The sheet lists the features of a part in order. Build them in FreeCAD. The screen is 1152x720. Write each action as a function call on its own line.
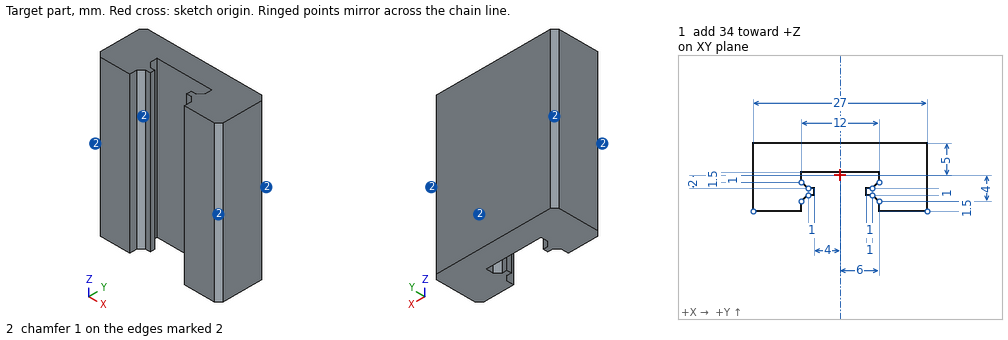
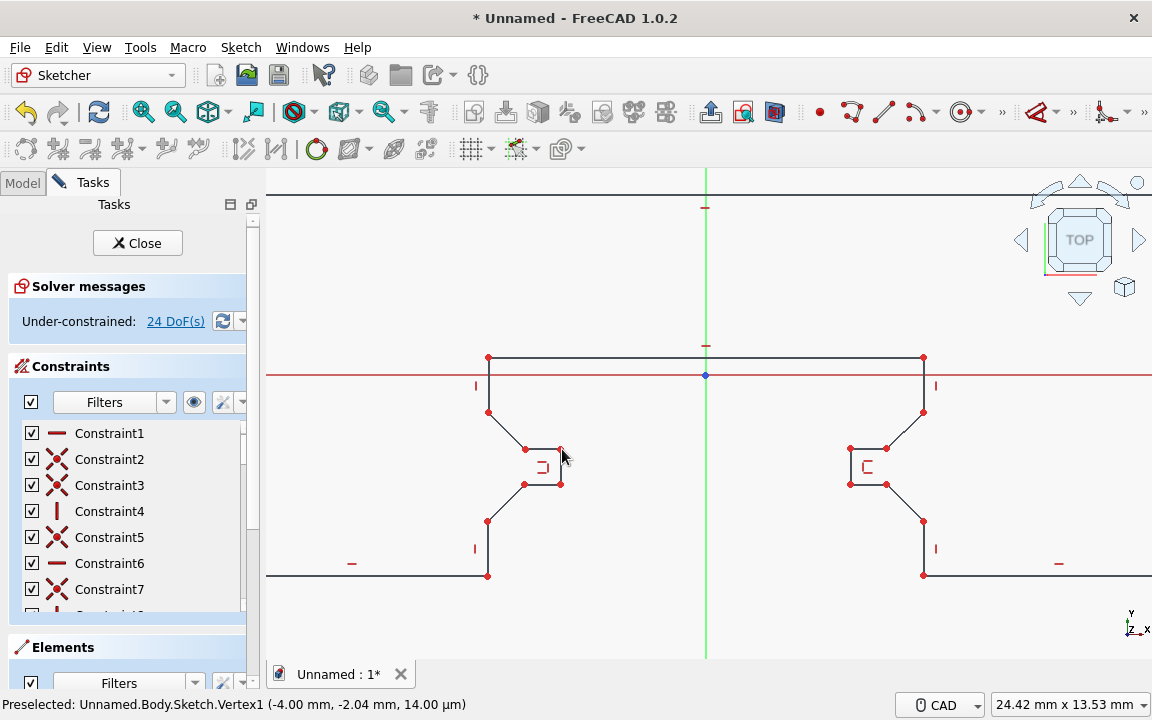
click(489, 413)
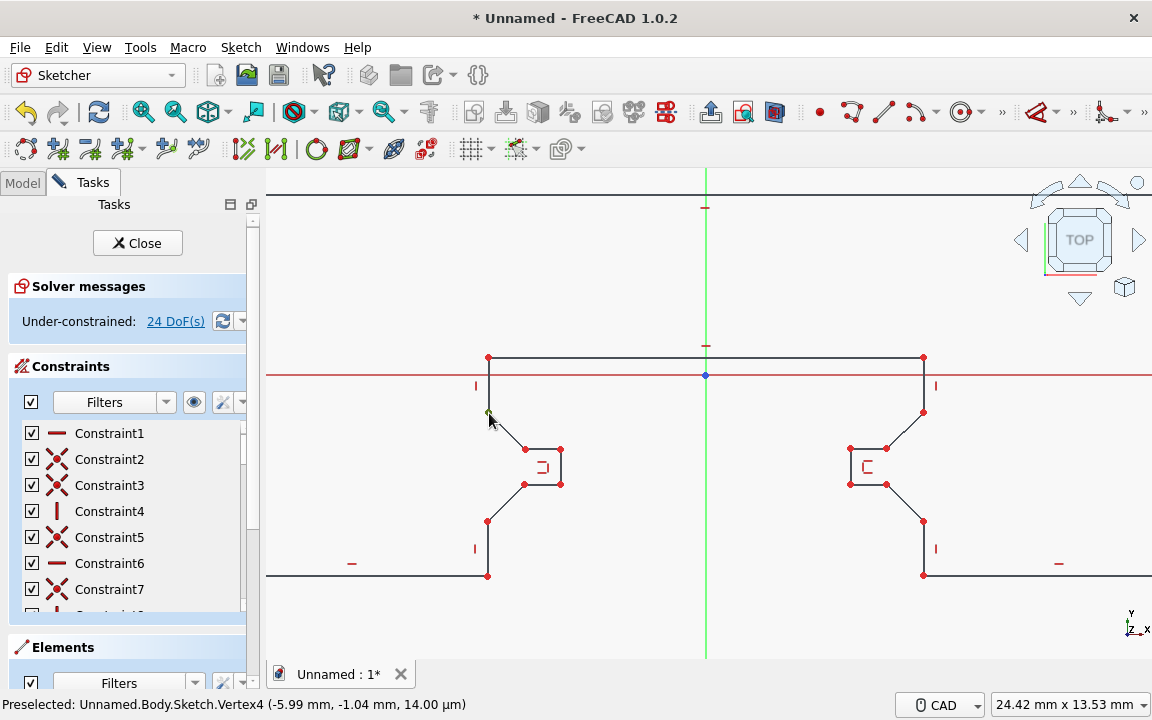
click(924, 413)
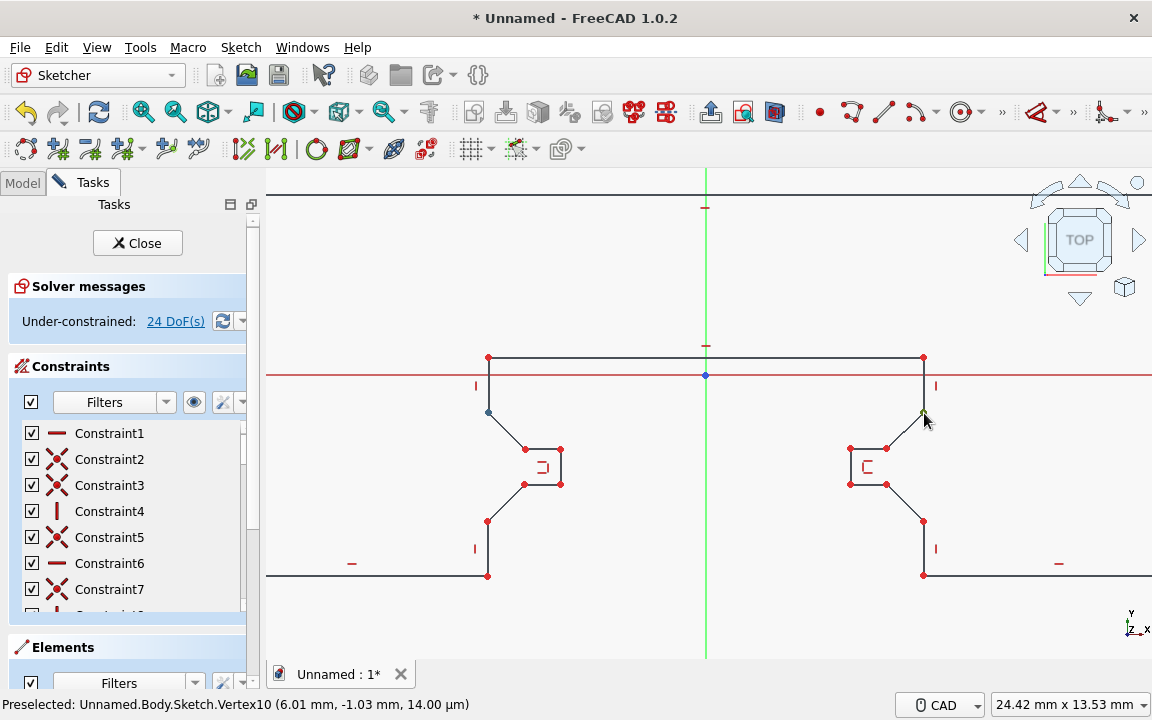
click(706, 600)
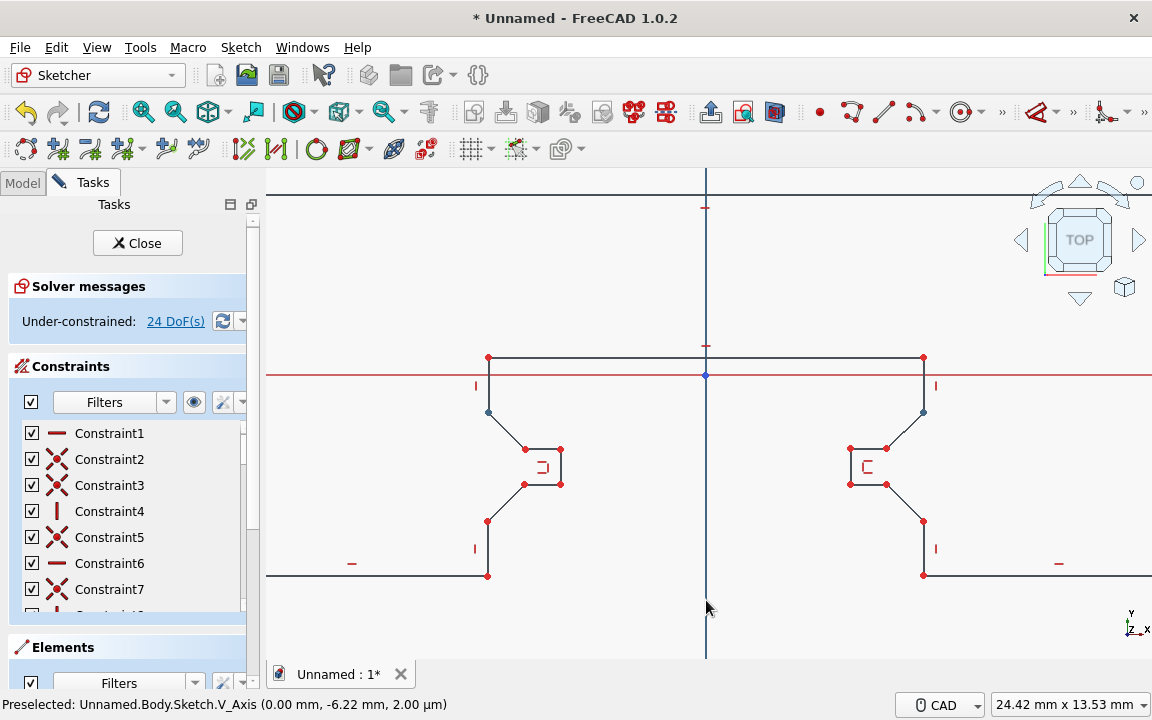
key(s)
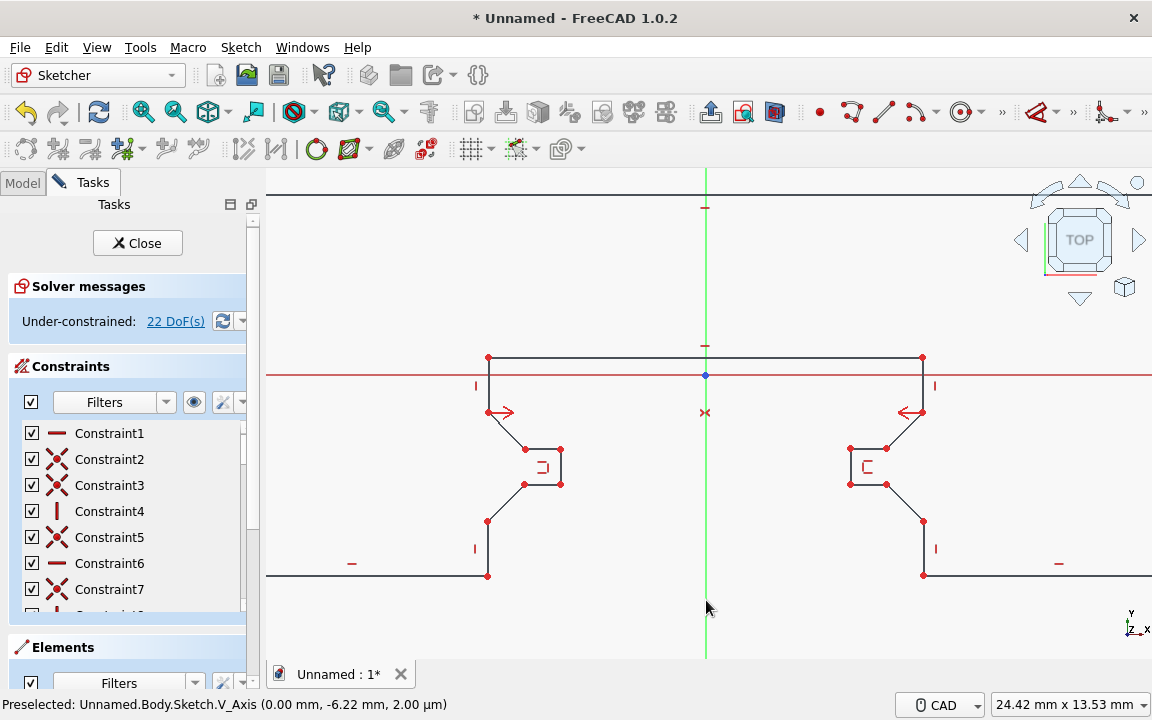
click(525, 449)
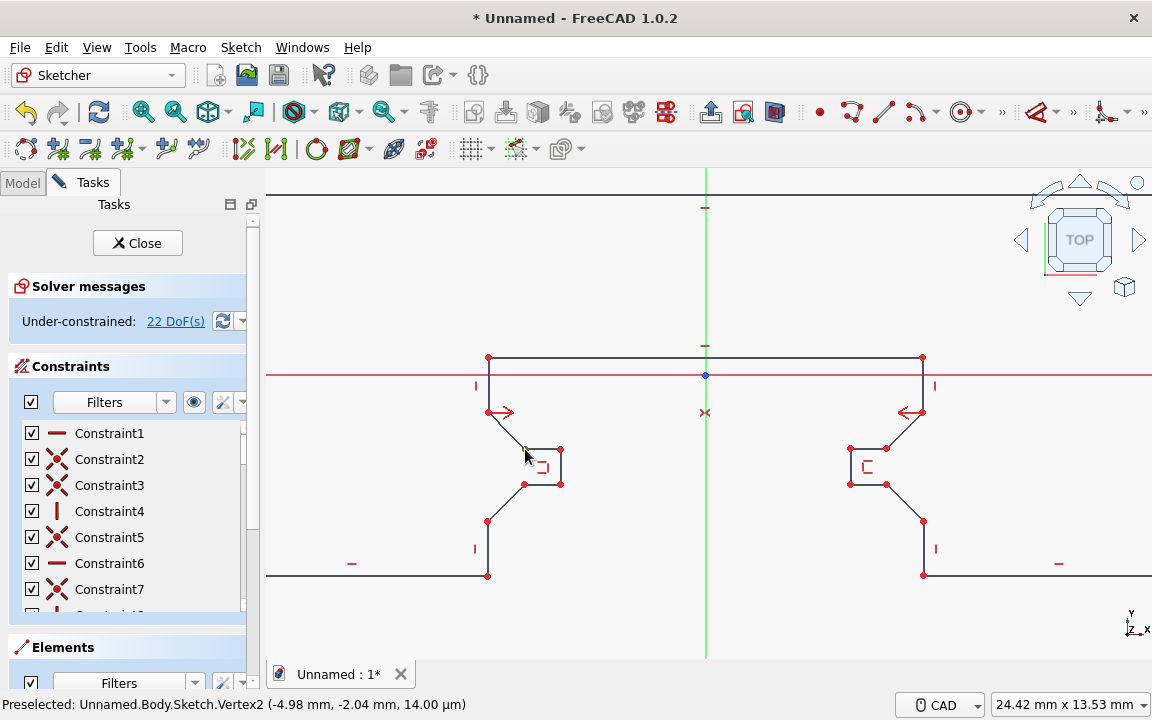
click(887, 449)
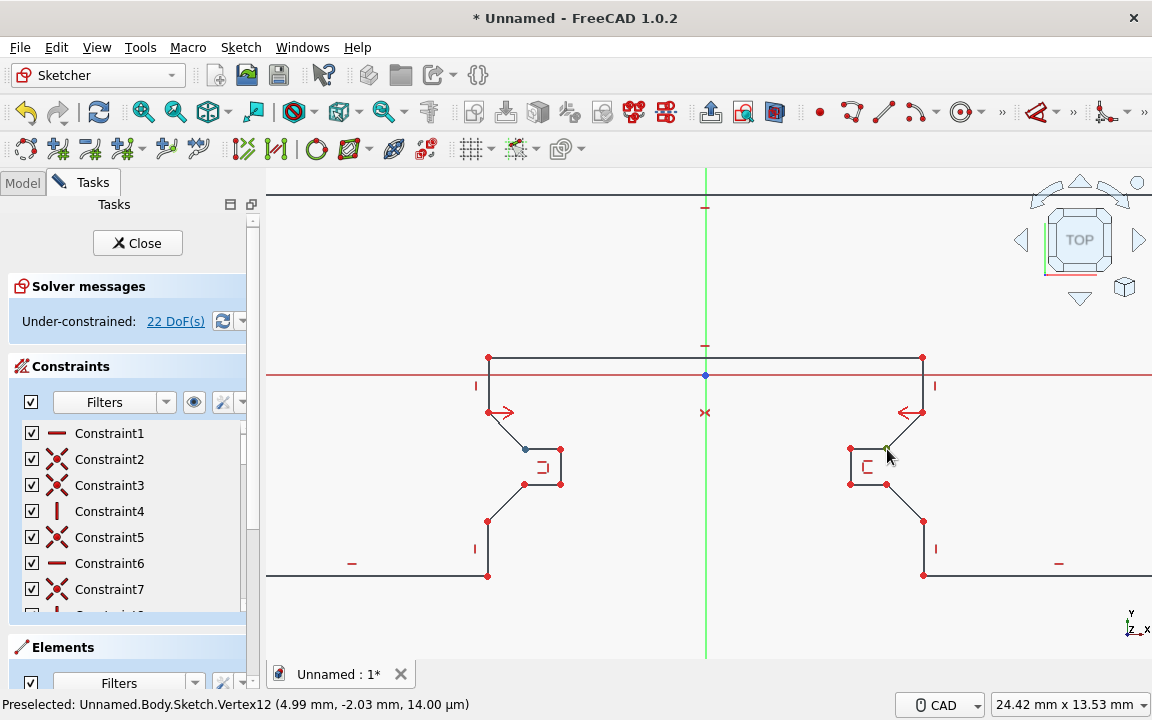
click(706, 600)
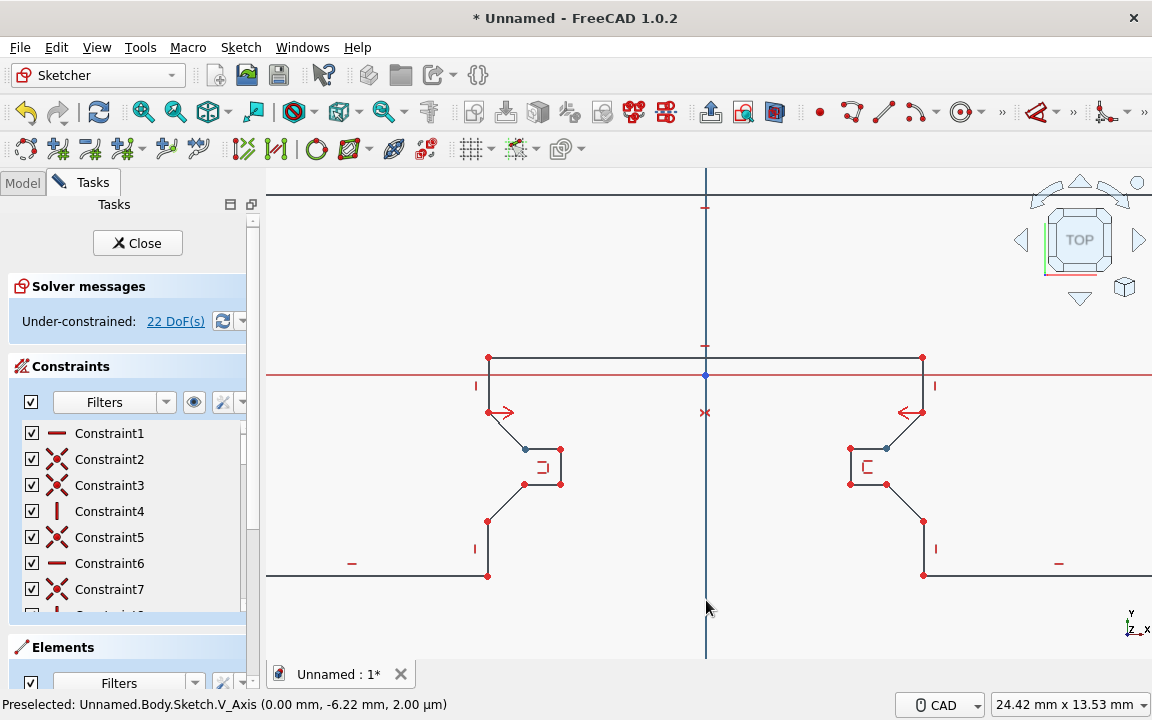
key(s)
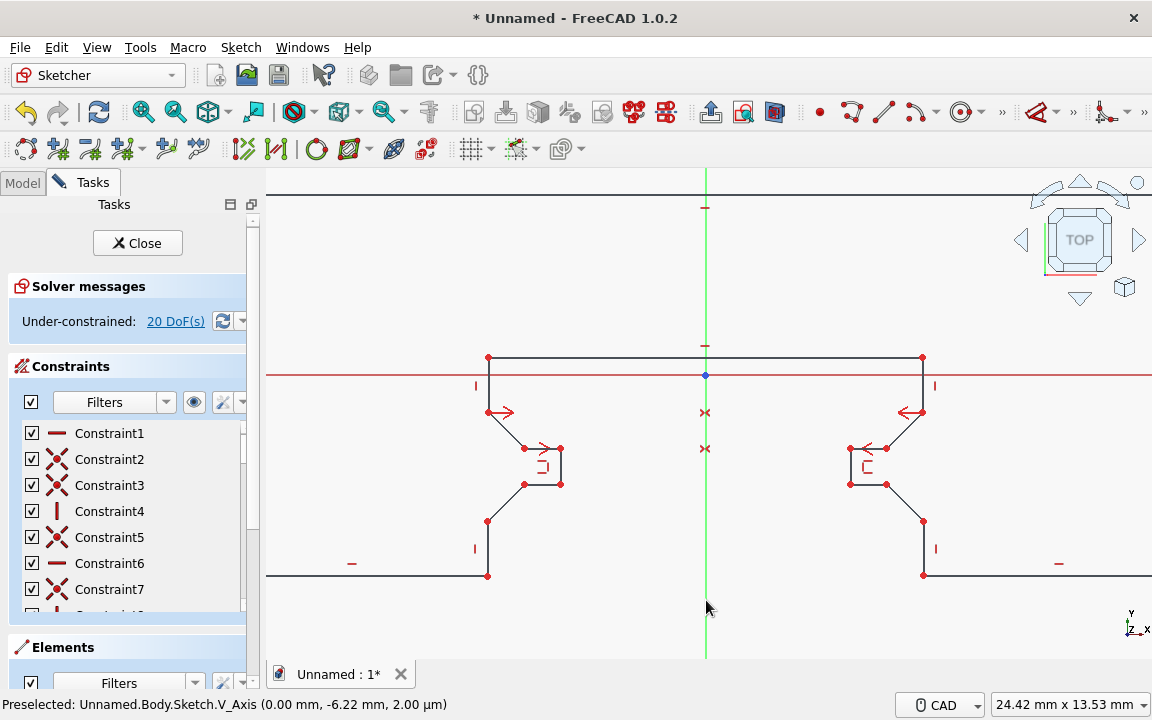
scroll(561, 449, down, 3)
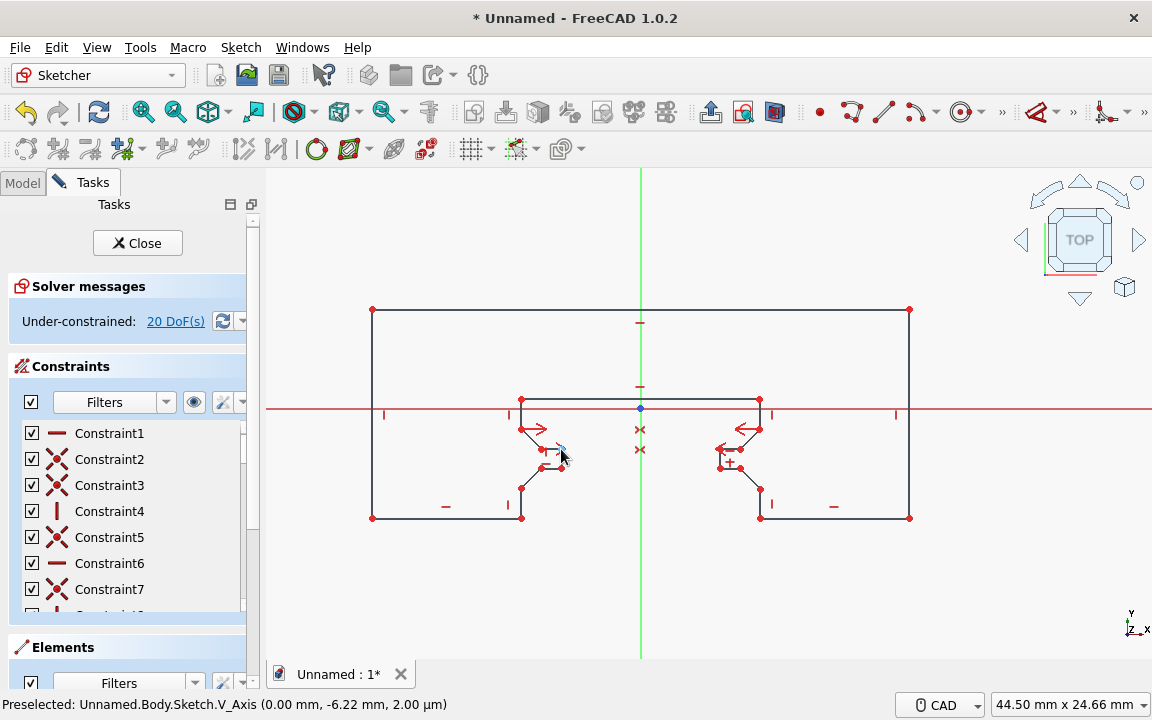
click(909, 519)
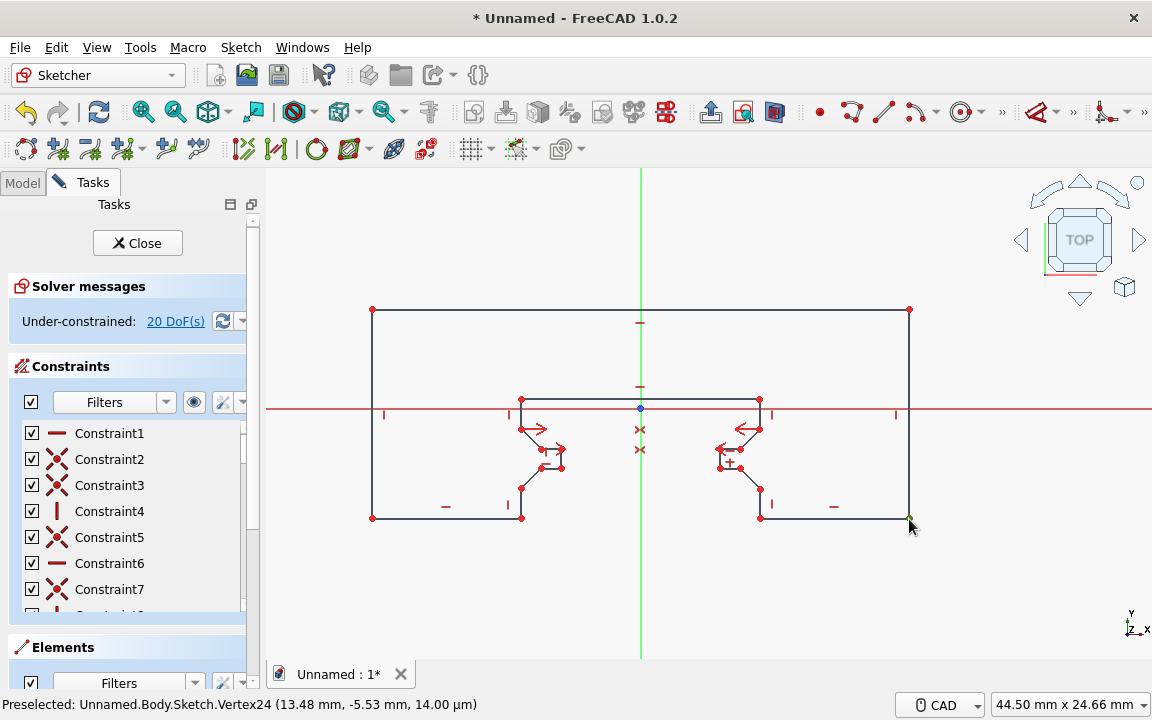
click(372, 519)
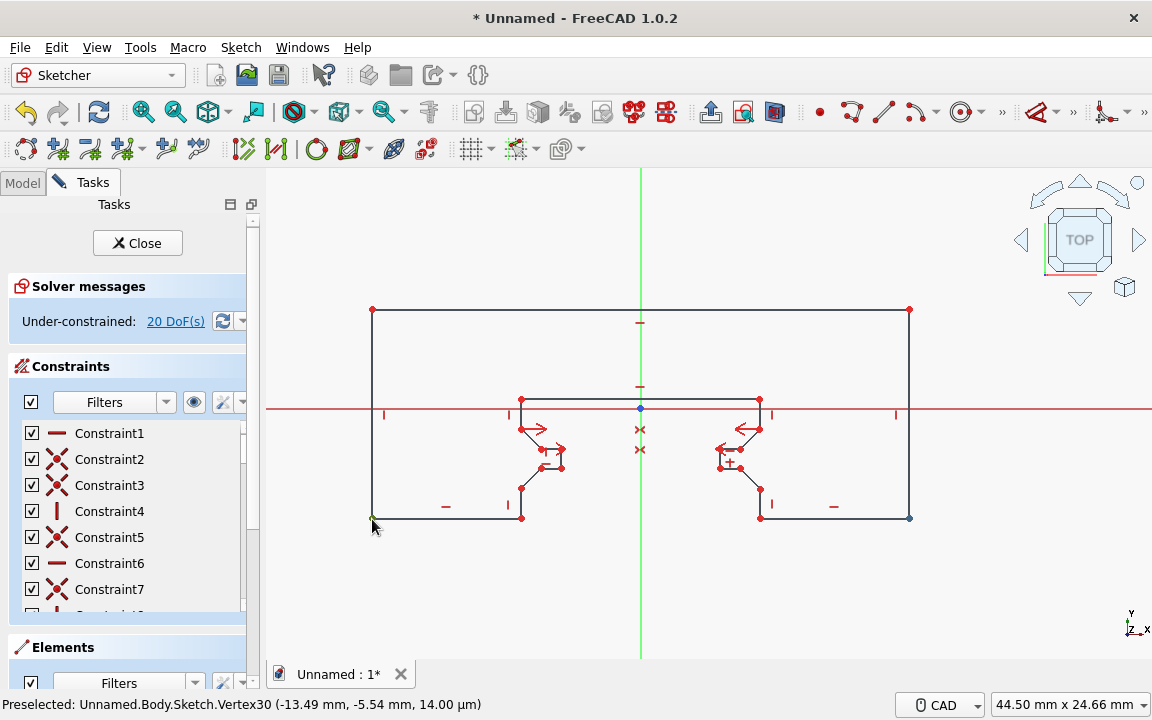
click(641, 600)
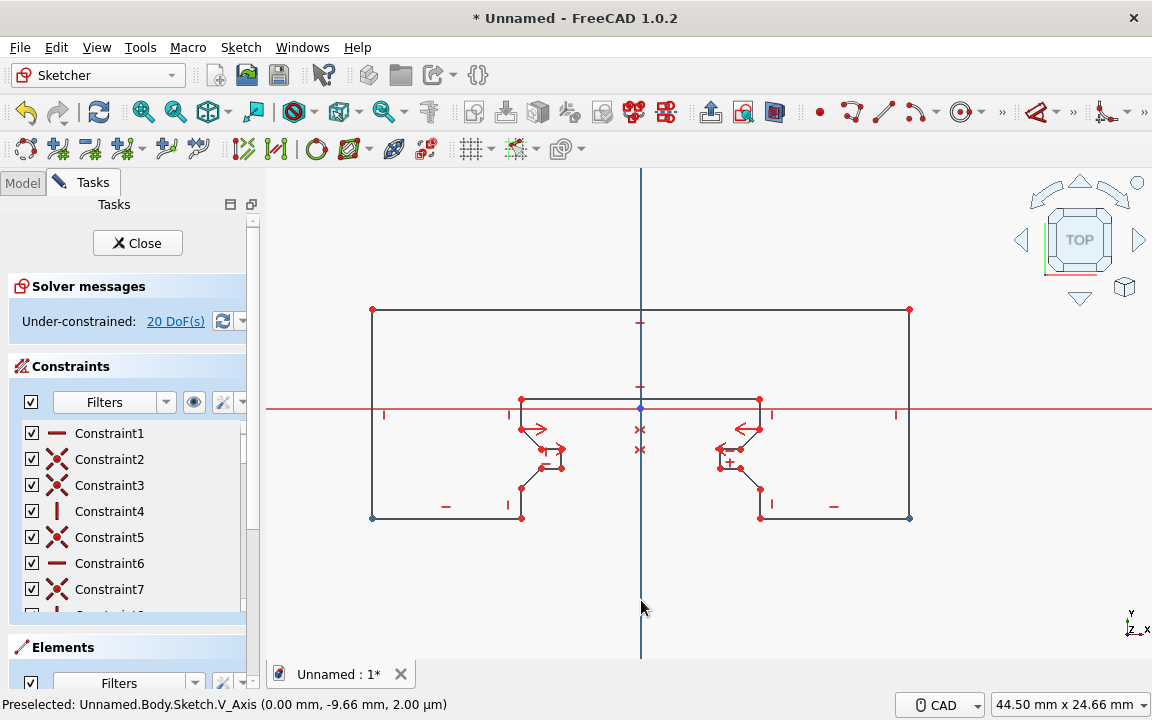
key(s)